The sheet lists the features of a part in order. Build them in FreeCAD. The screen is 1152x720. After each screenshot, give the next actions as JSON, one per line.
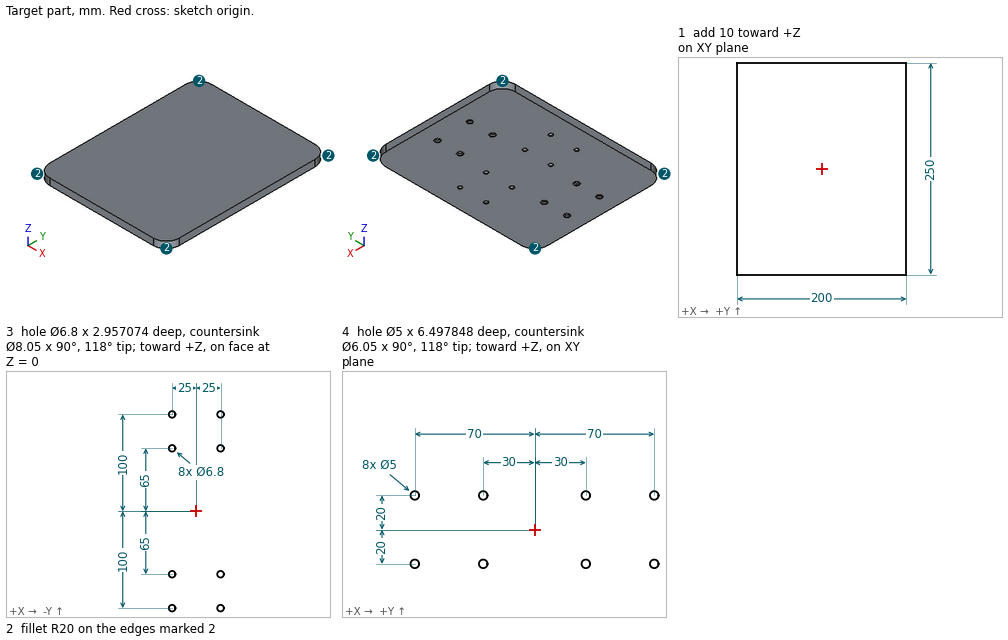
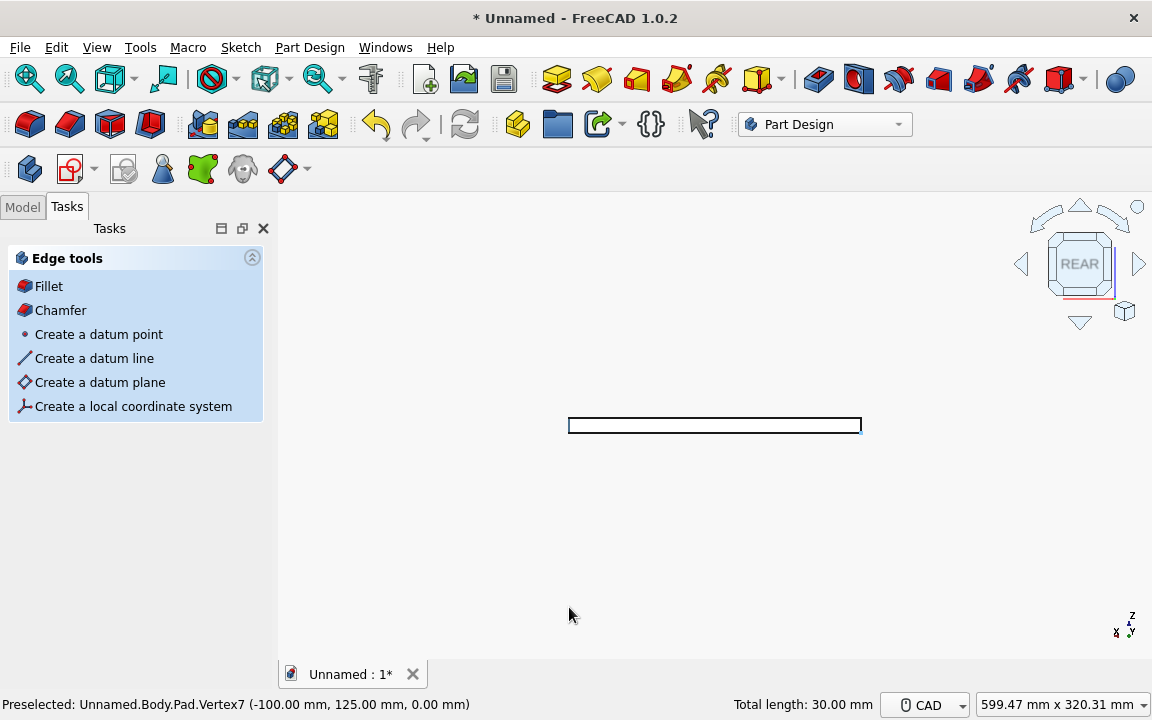
{"action": "left_click", "coordinate": [30, 80]}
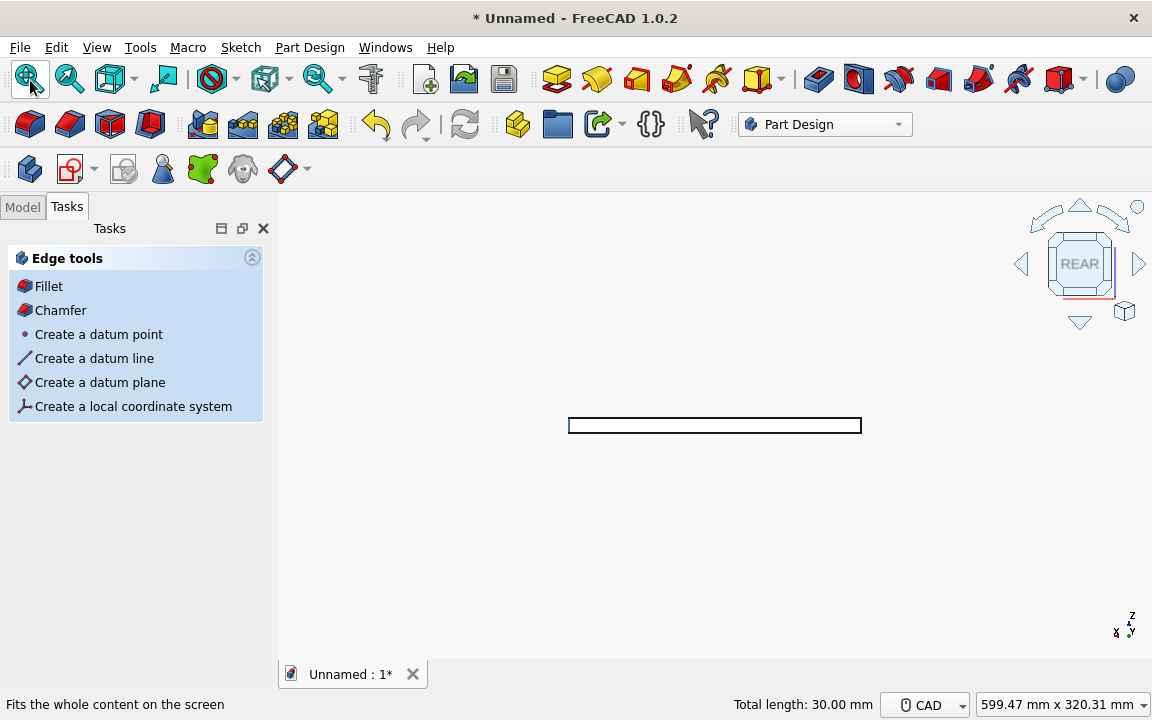
{"action": "left_click", "coordinate": [861, 425], "text": "ctrl"}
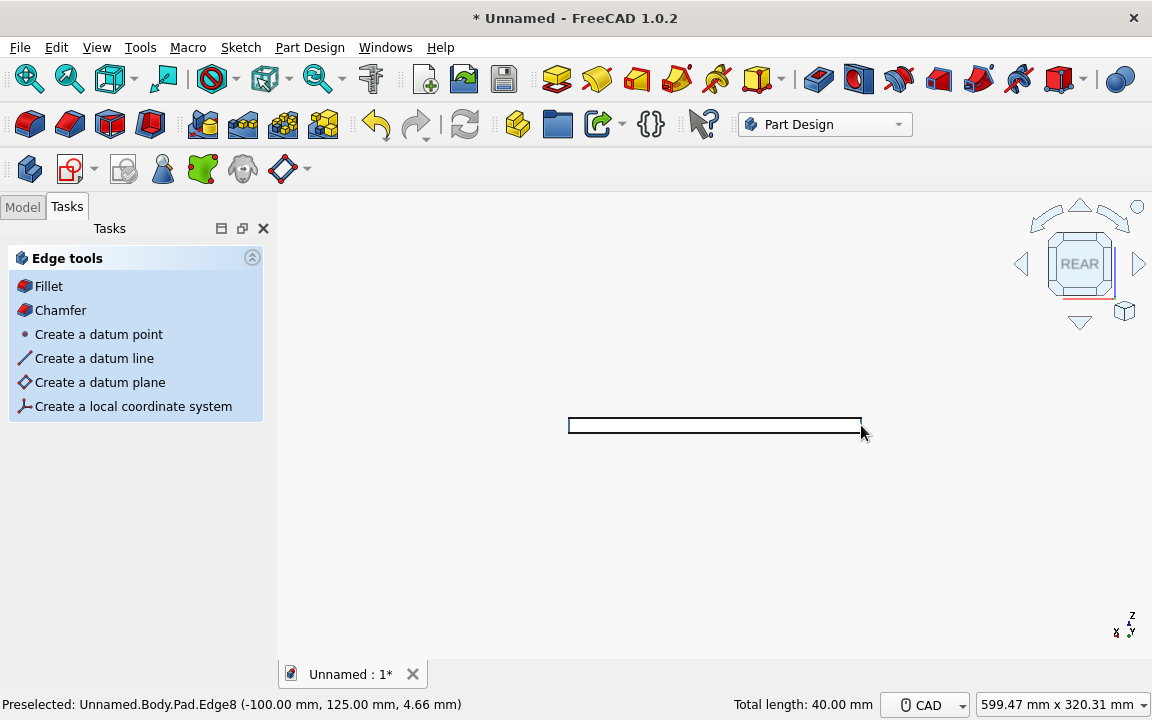
{"action": "left_click", "coordinate": [30, 124]}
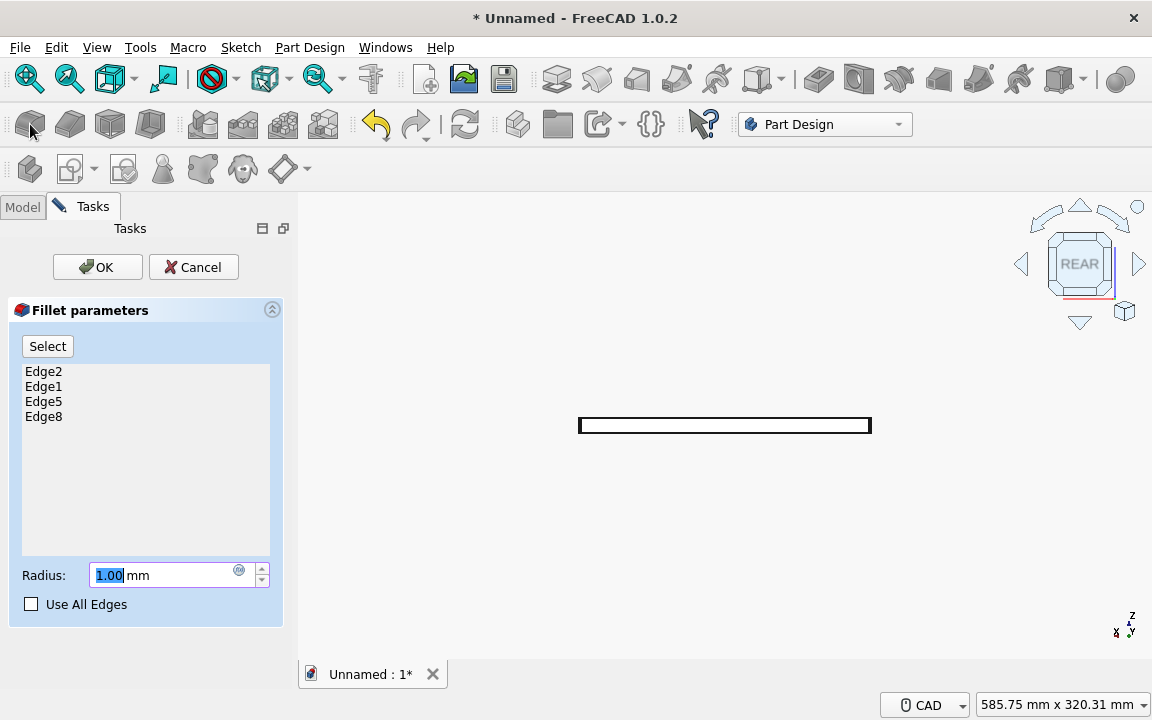
{"action": "type", "text": "20"}
{"action": "key", "text": "Tab"}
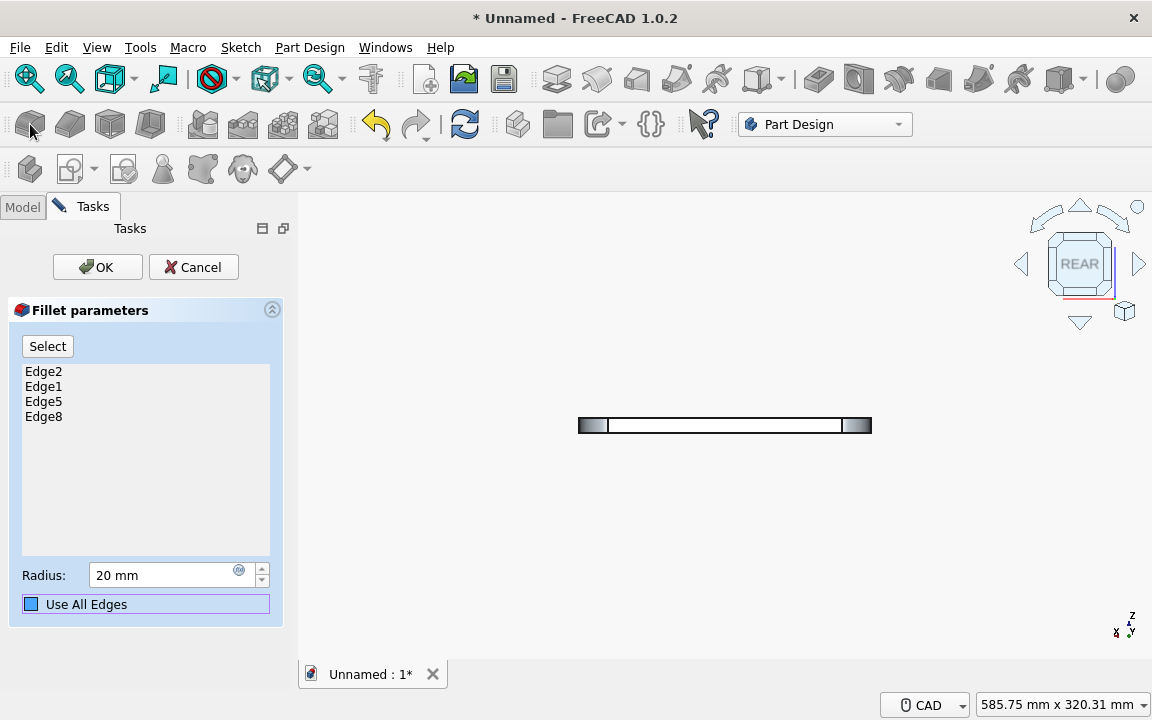
{"action": "left_click", "coordinate": [98, 267]}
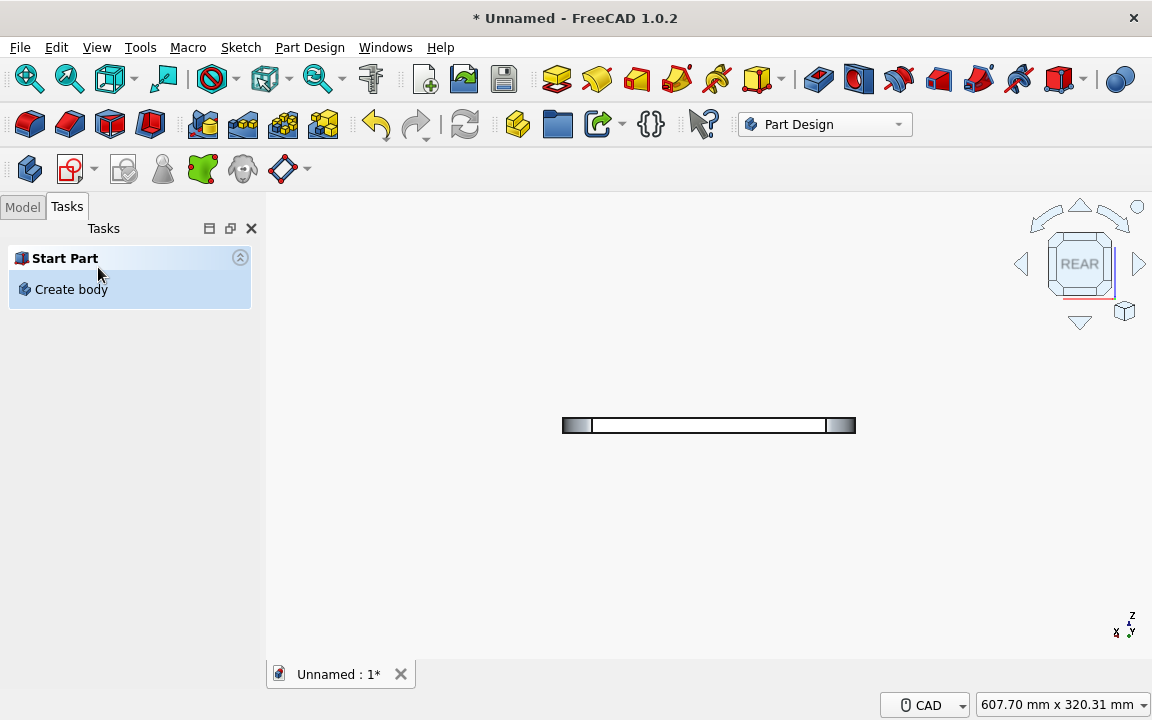
{"action": "key", "text": "v f"}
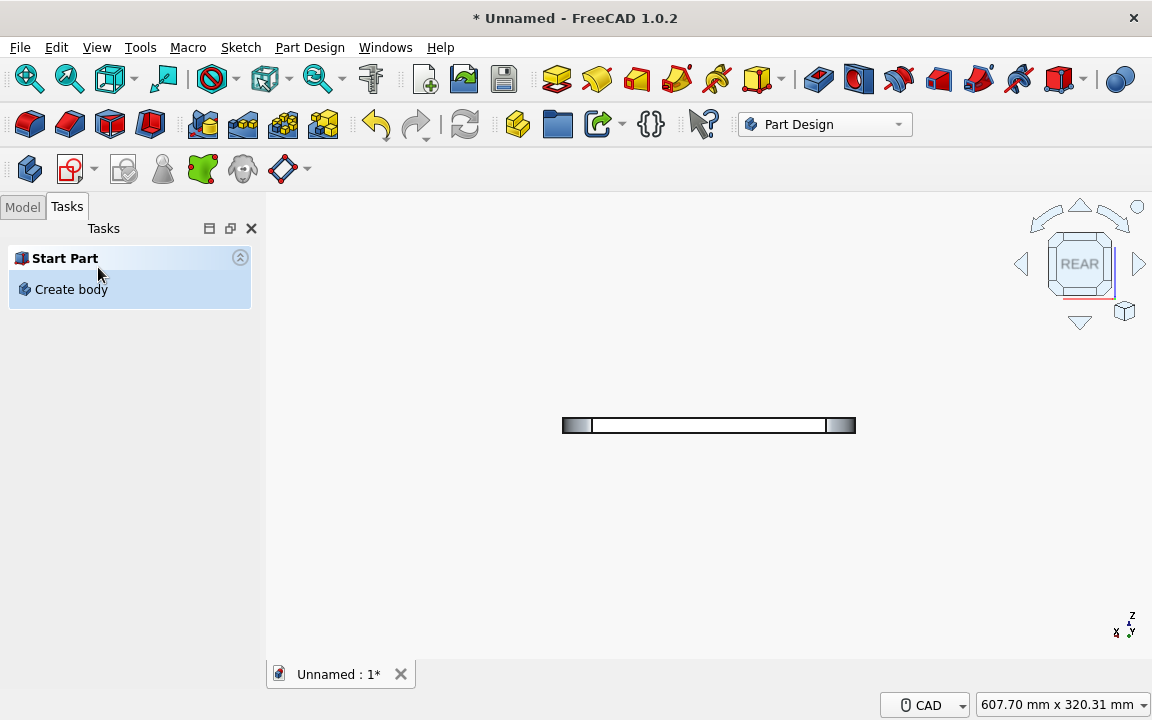
{"action": "key", "text": "5"}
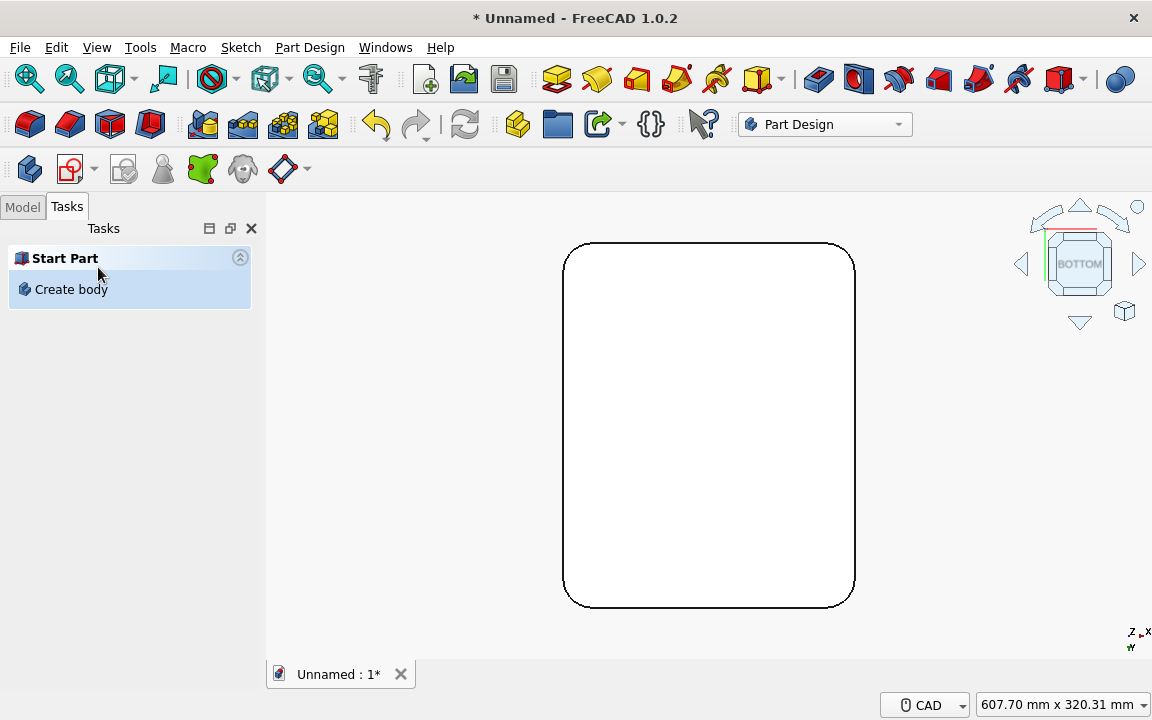
{"action": "left_click", "coordinate": [709, 424]}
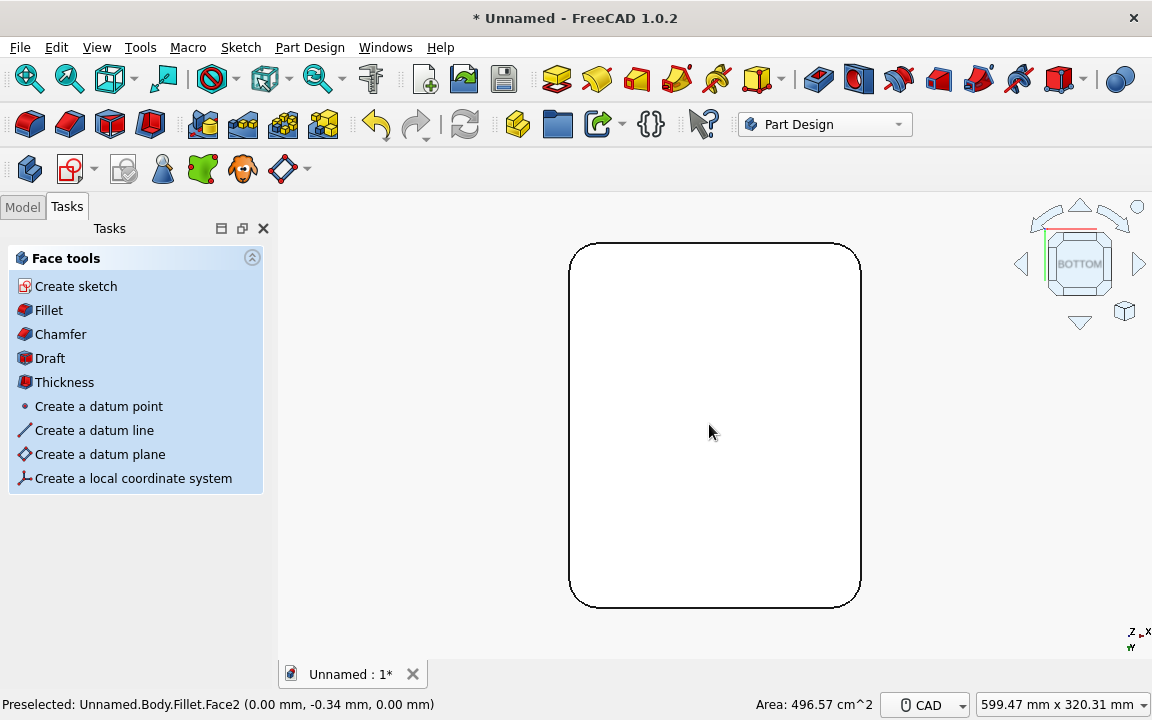
{"action": "left_click", "coordinate": [70, 170]}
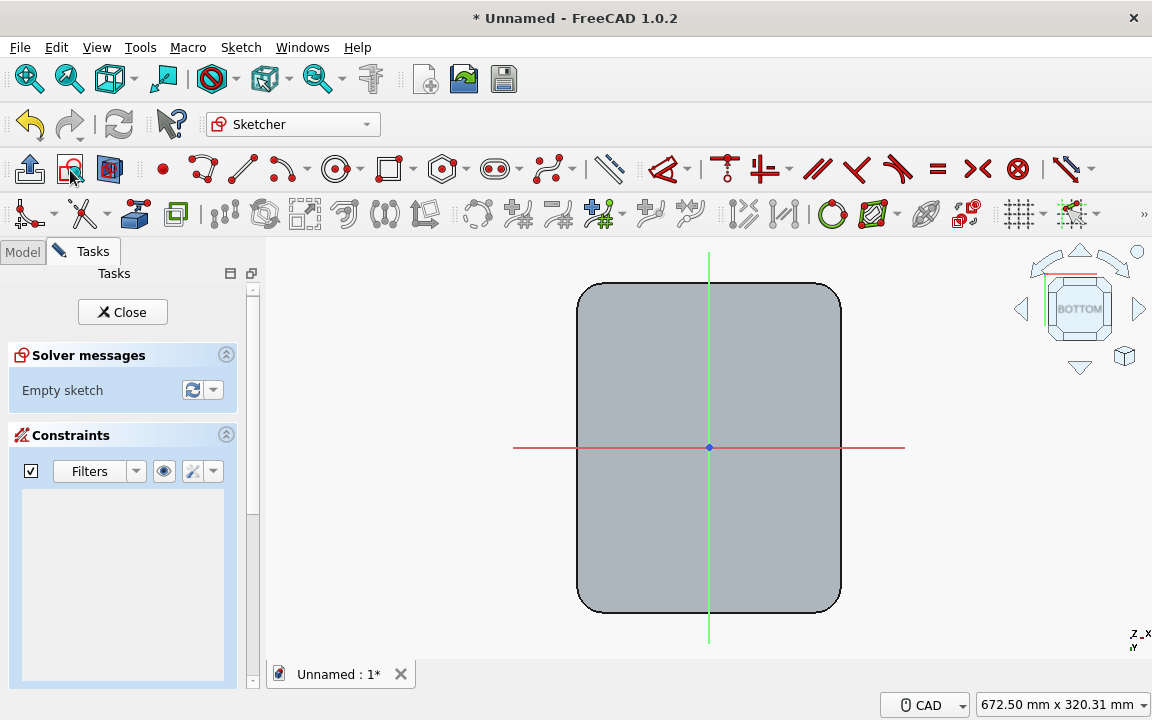
{"action": "left_click", "coordinate": [336, 170]}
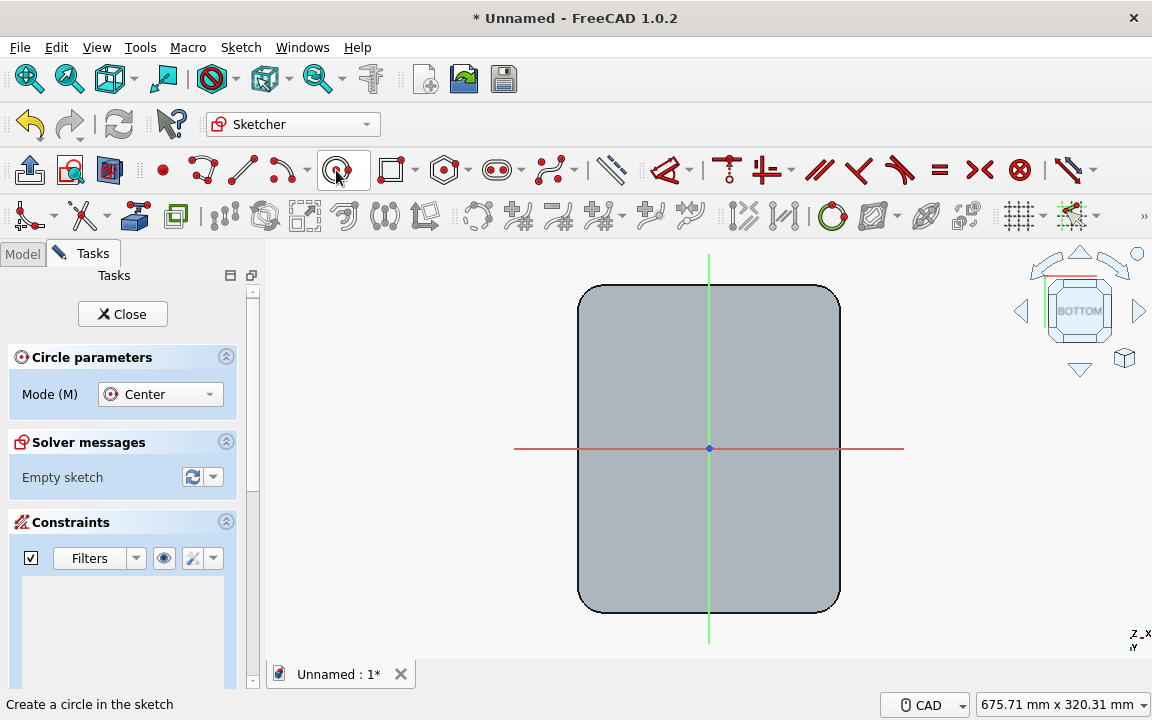
{"action": "scroll", "coordinate": [676, 318], "scroll_direction": "up", "scroll_amount": 9}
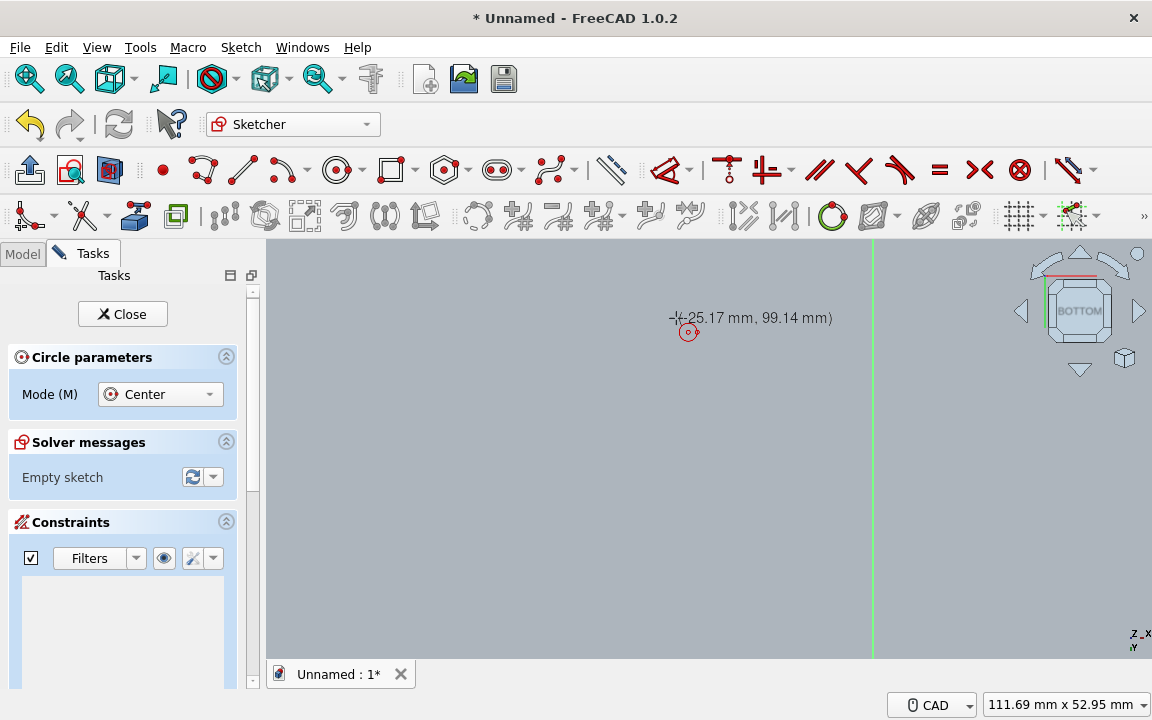
{"action": "scroll", "coordinate": [594, 318], "scroll_direction": "down", "scroll_amount": 9}